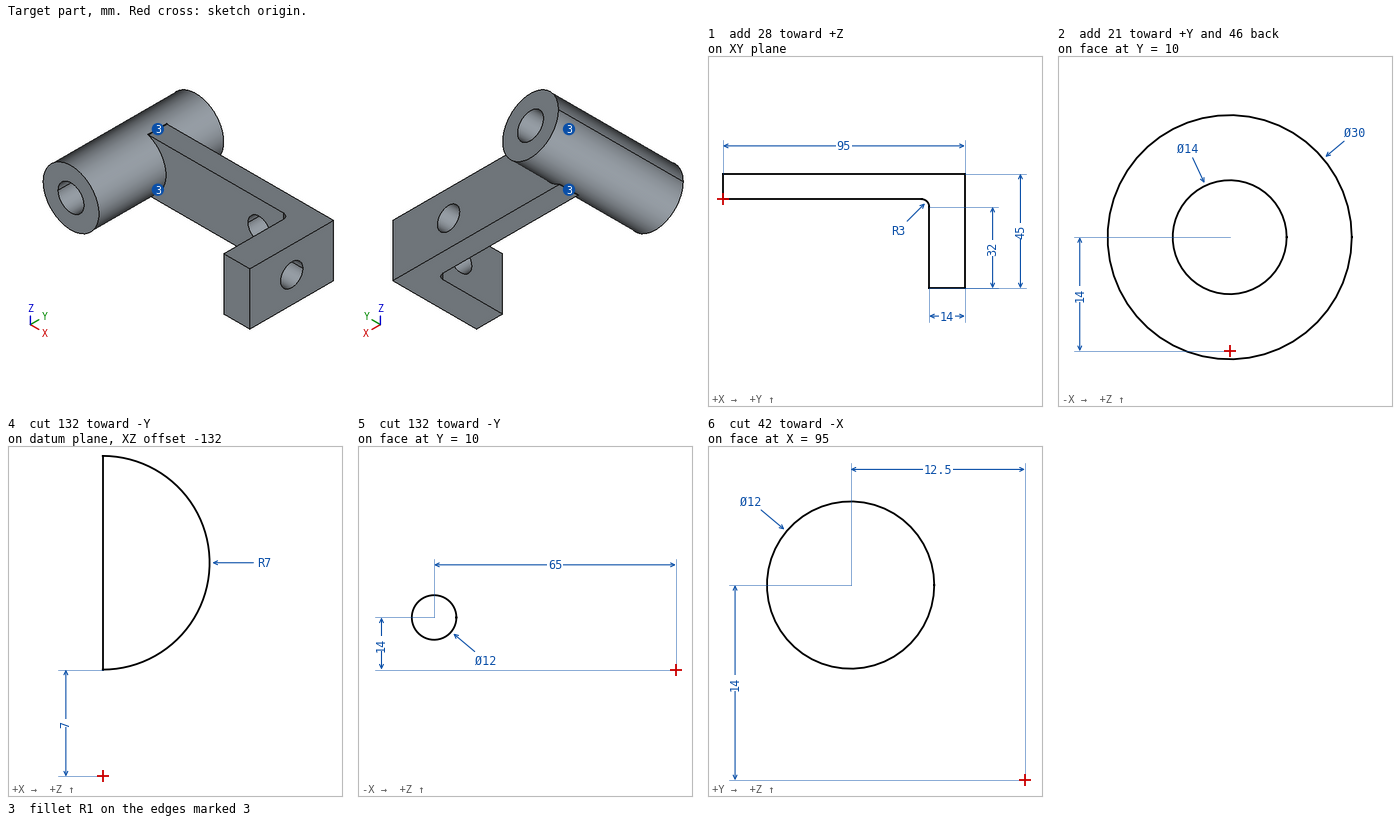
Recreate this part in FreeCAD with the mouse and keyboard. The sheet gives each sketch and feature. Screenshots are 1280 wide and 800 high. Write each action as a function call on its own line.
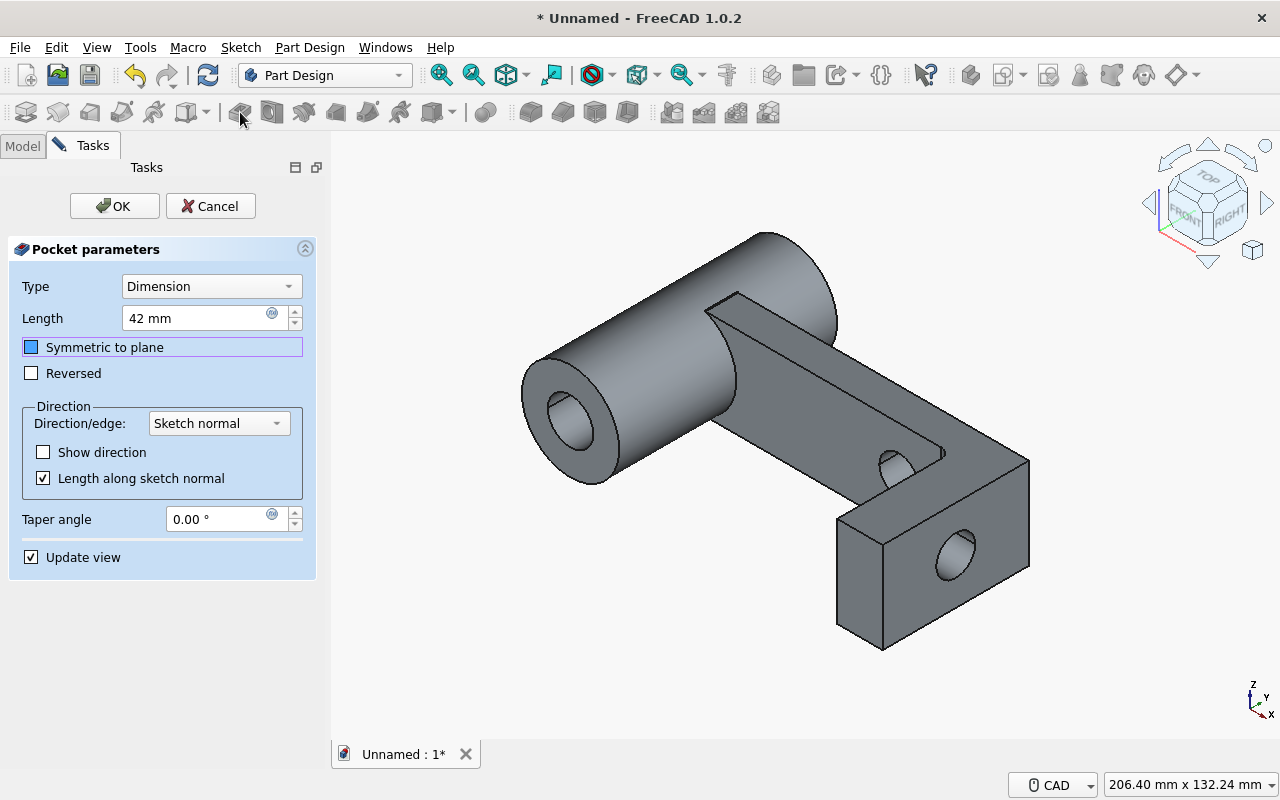
click(115, 206)